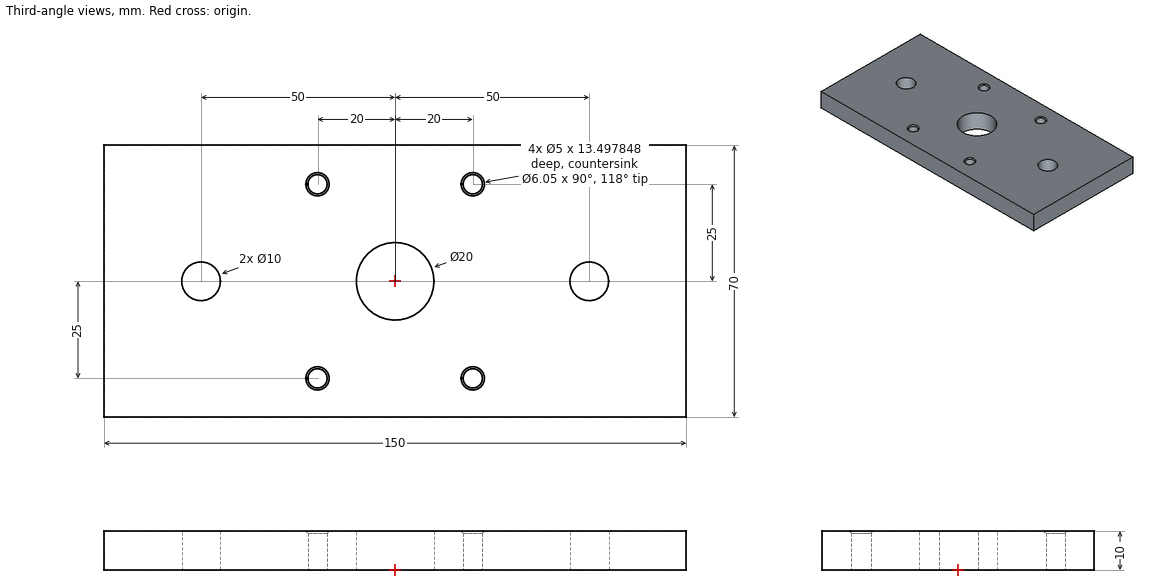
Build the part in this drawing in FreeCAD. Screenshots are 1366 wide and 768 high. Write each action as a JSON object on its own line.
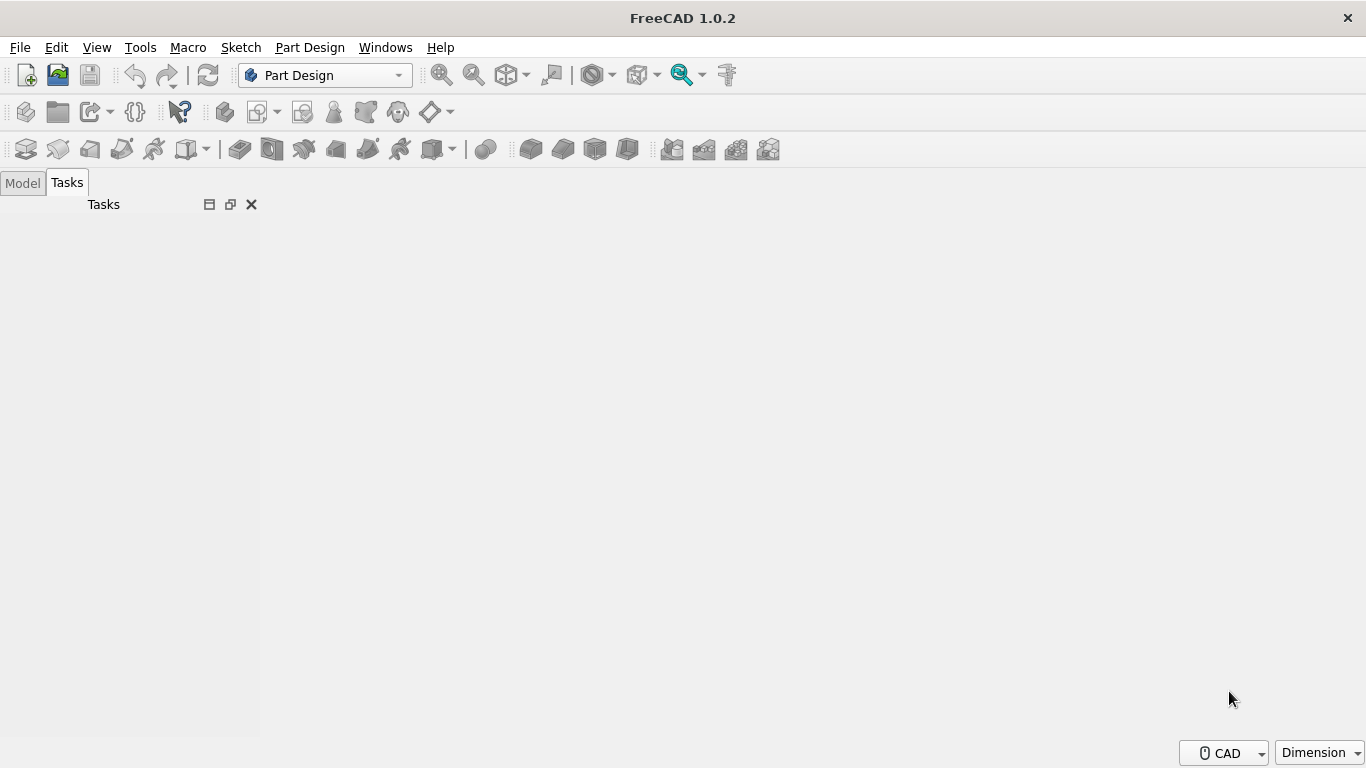
{"action": "left_click", "coordinate": [26, 76]}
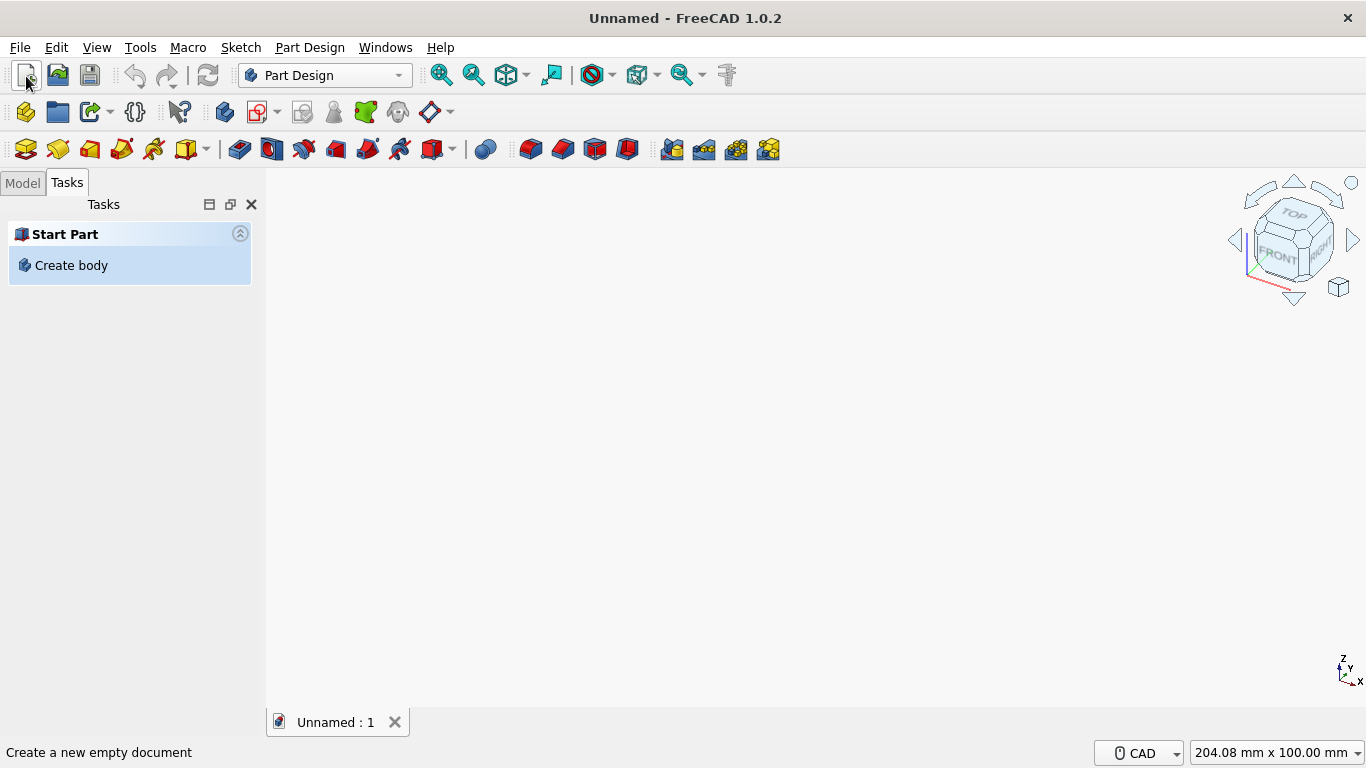
{"action": "left_click", "coordinate": [258, 112]}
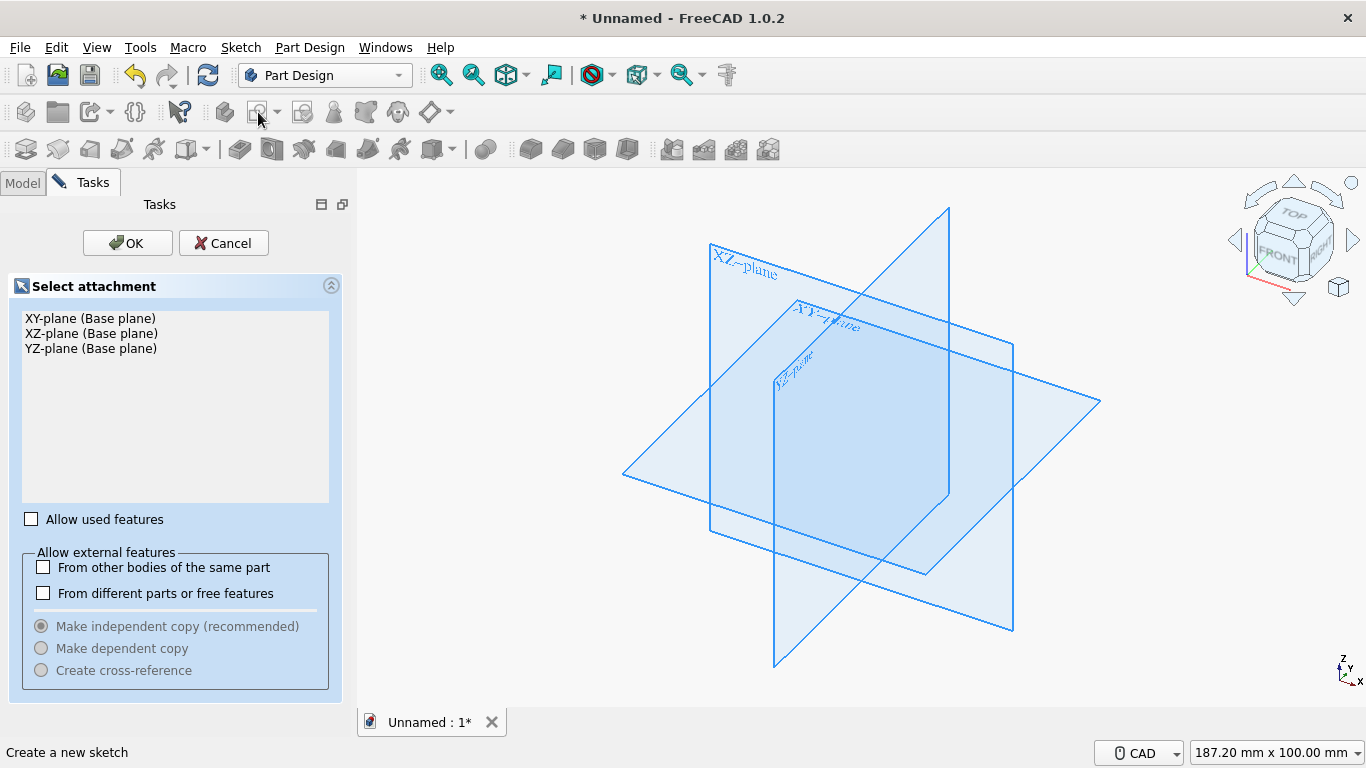
{"action": "left_click", "coordinate": [82, 318]}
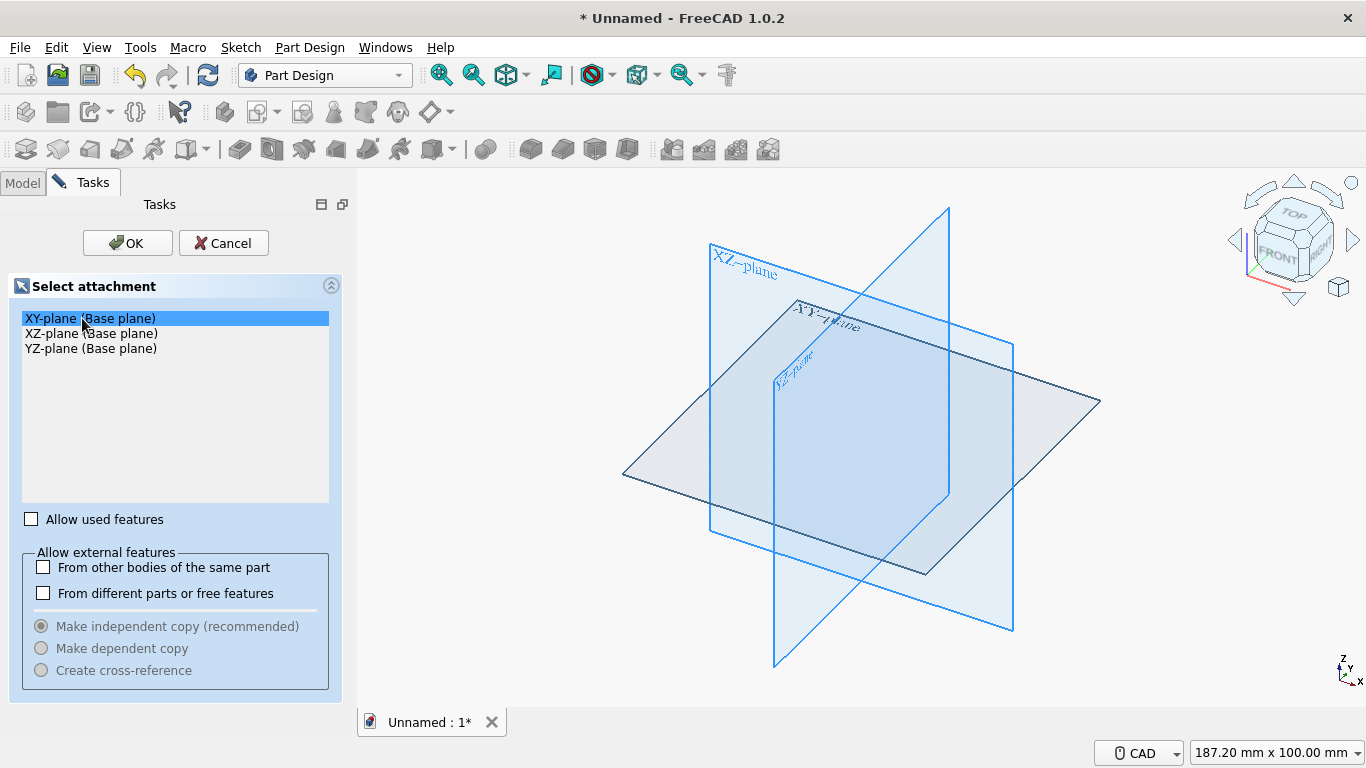
{"action": "left_click", "coordinate": [128, 243]}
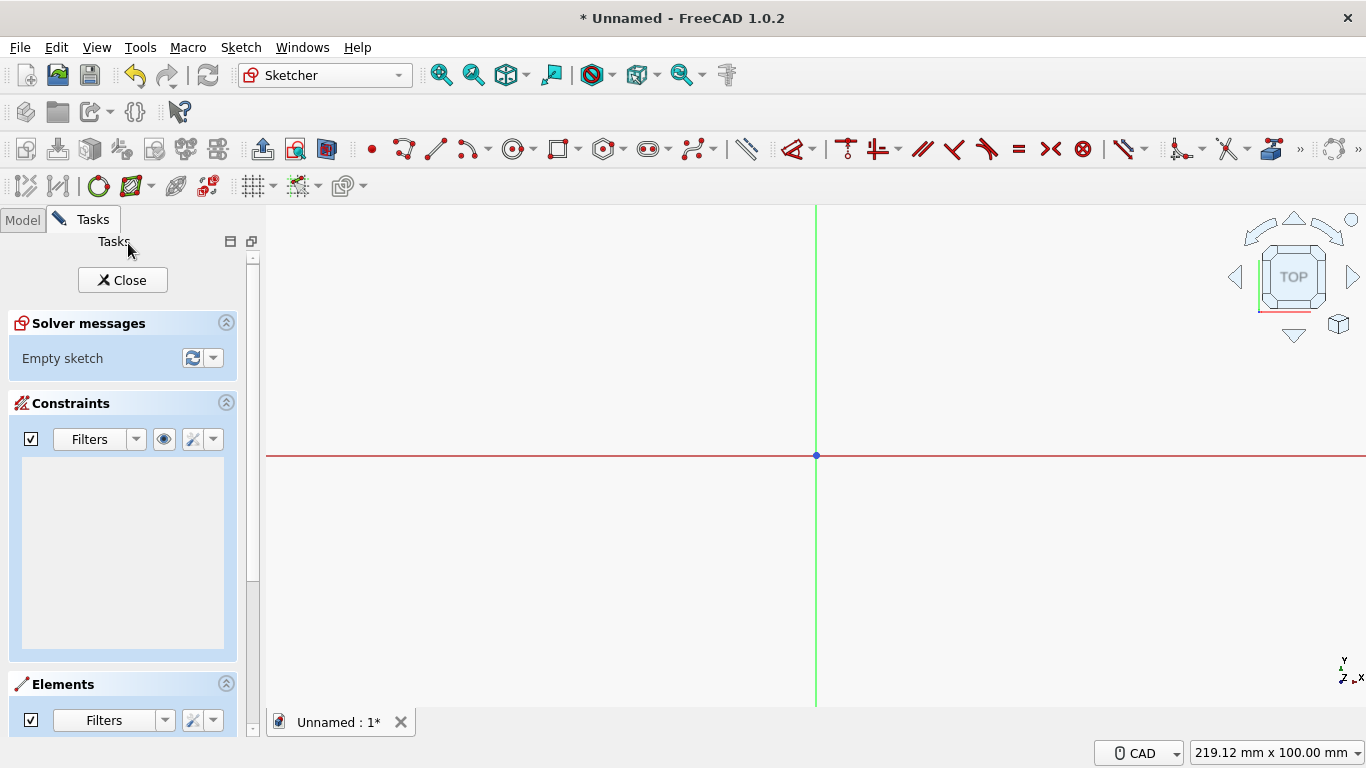
{"action": "scroll", "coordinate": [438, 456], "scroll_direction": "down", "scroll_amount": 1}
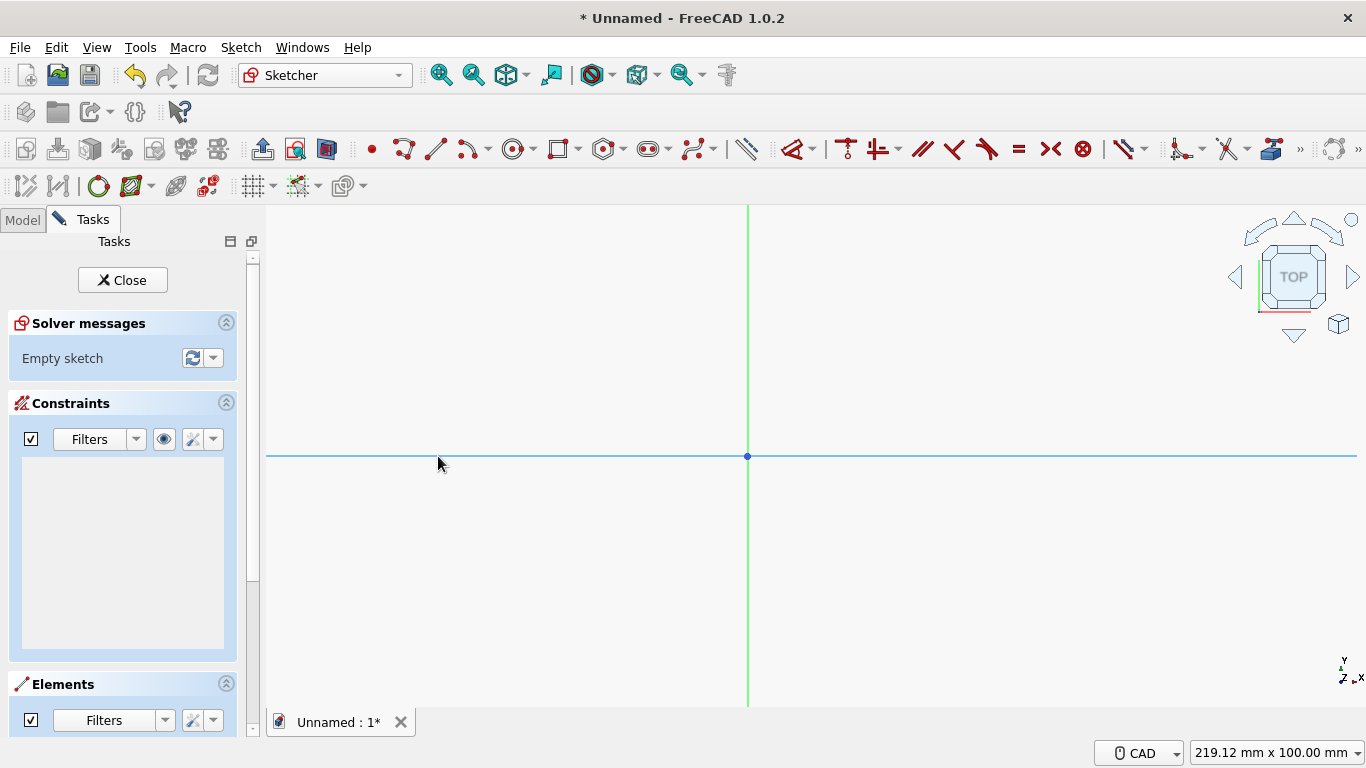
{"action": "left_click", "coordinate": [580, 150]}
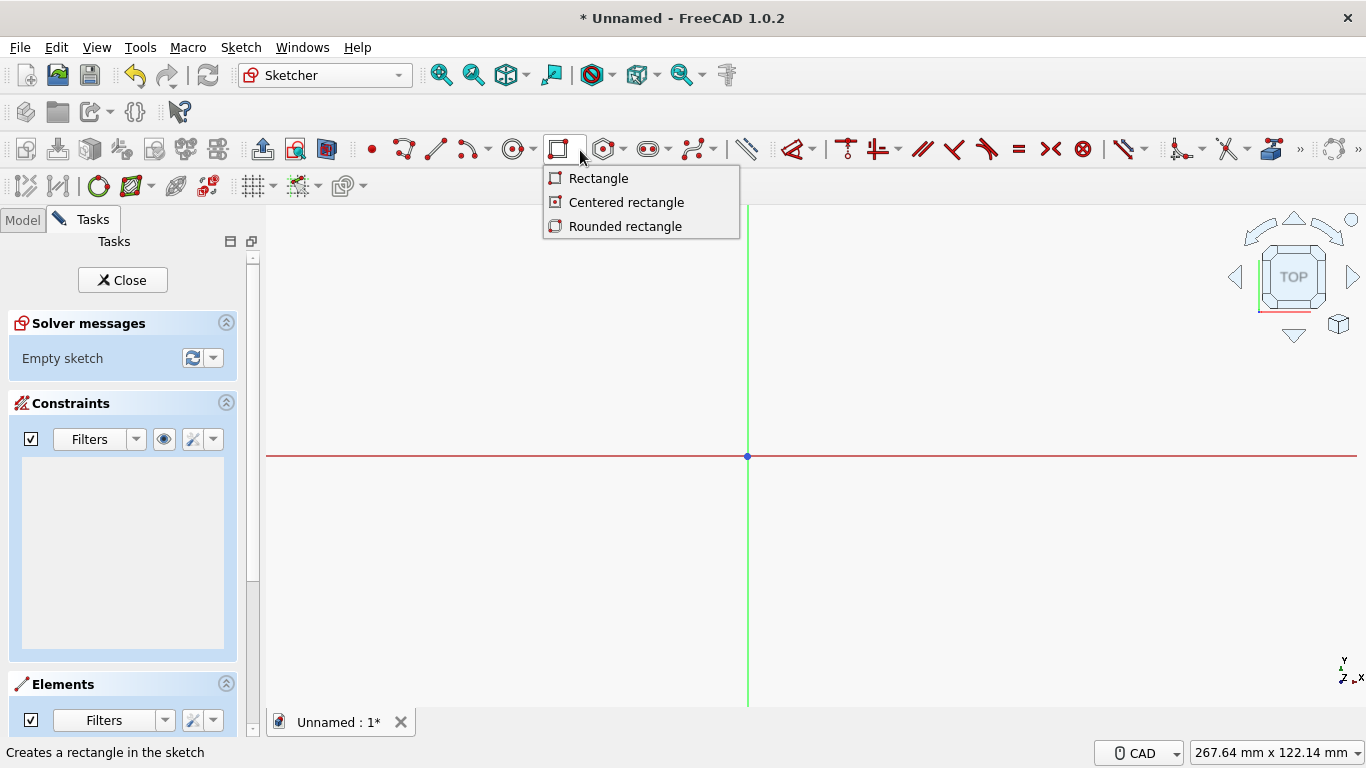
{"action": "left_click", "coordinate": [642, 202]}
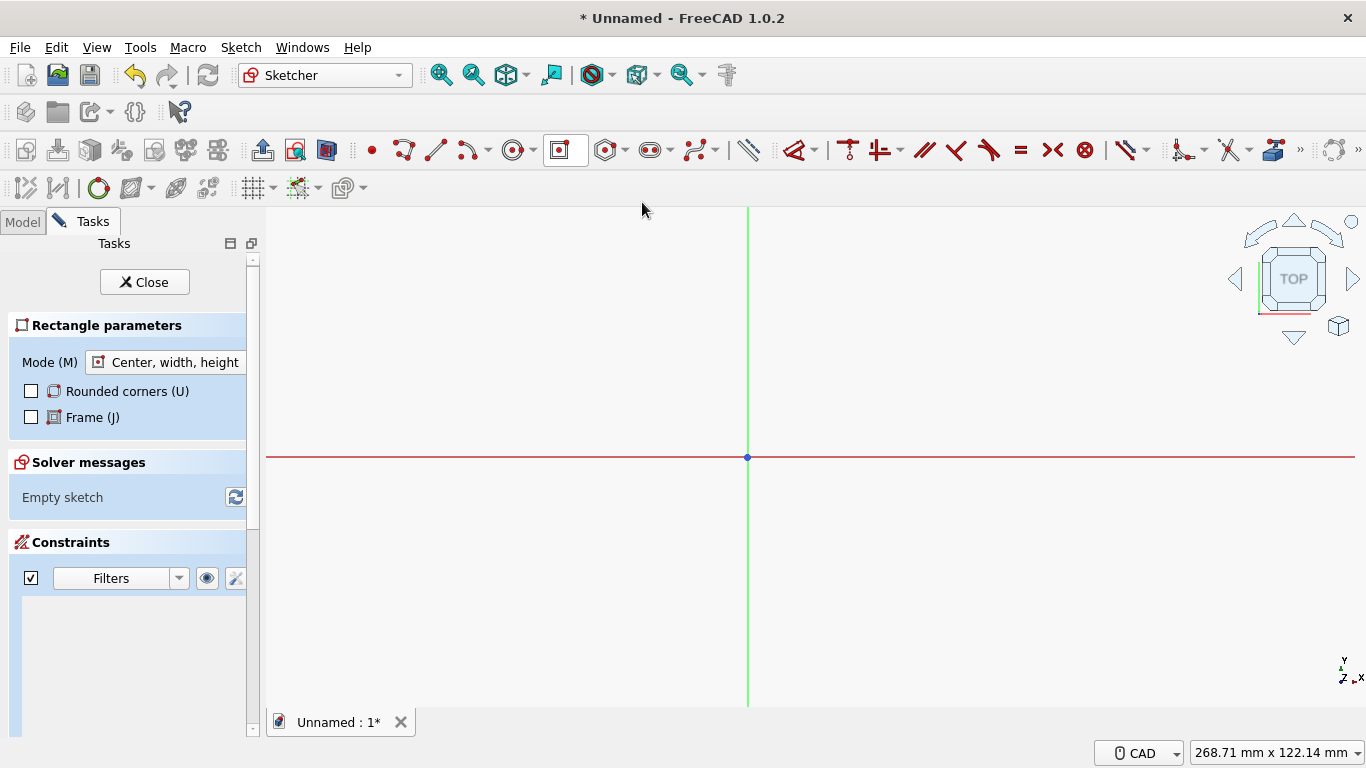
{"action": "left_click", "coordinate": [748, 457]}
{"action": "left_click", "coordinate": [1055, 314]}
{"action": "key", "text": "Escape"}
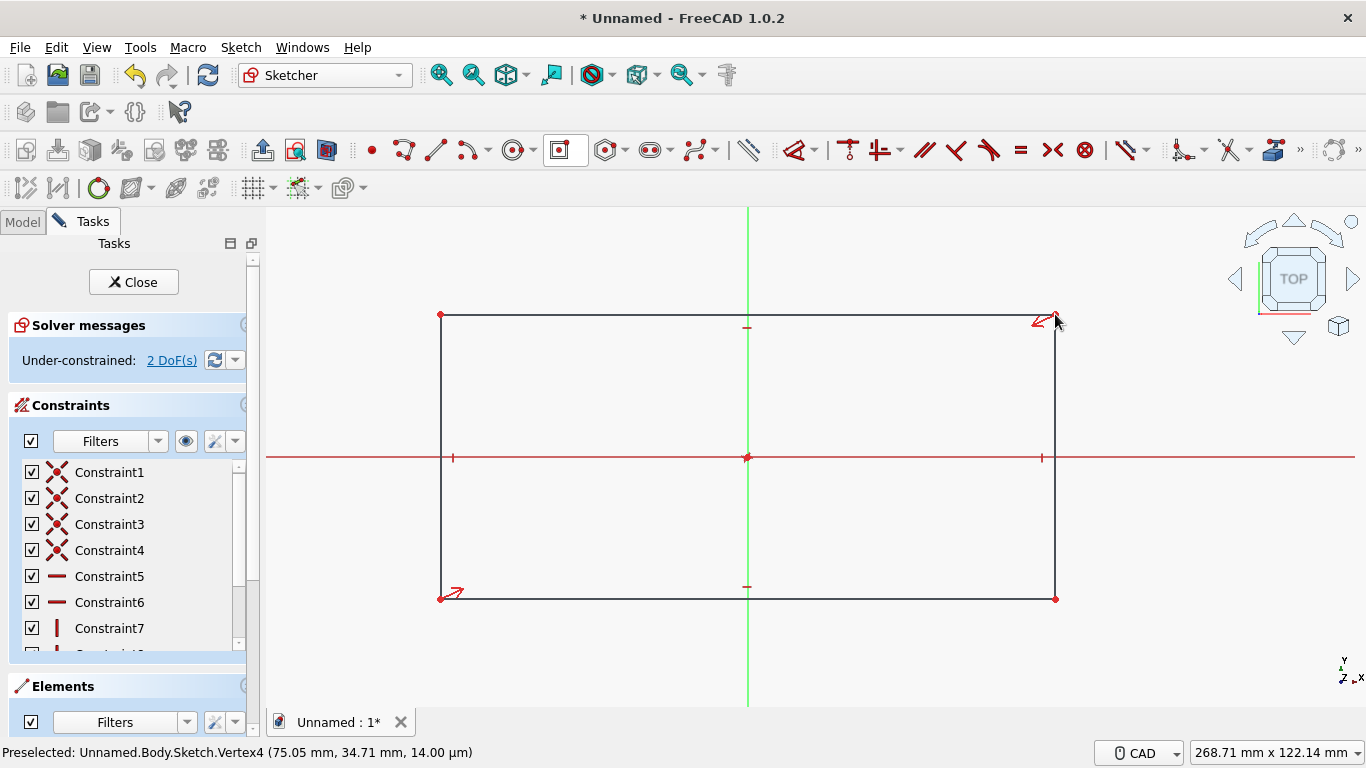
{"action": "left_click", "coordinate": [1055, 514]}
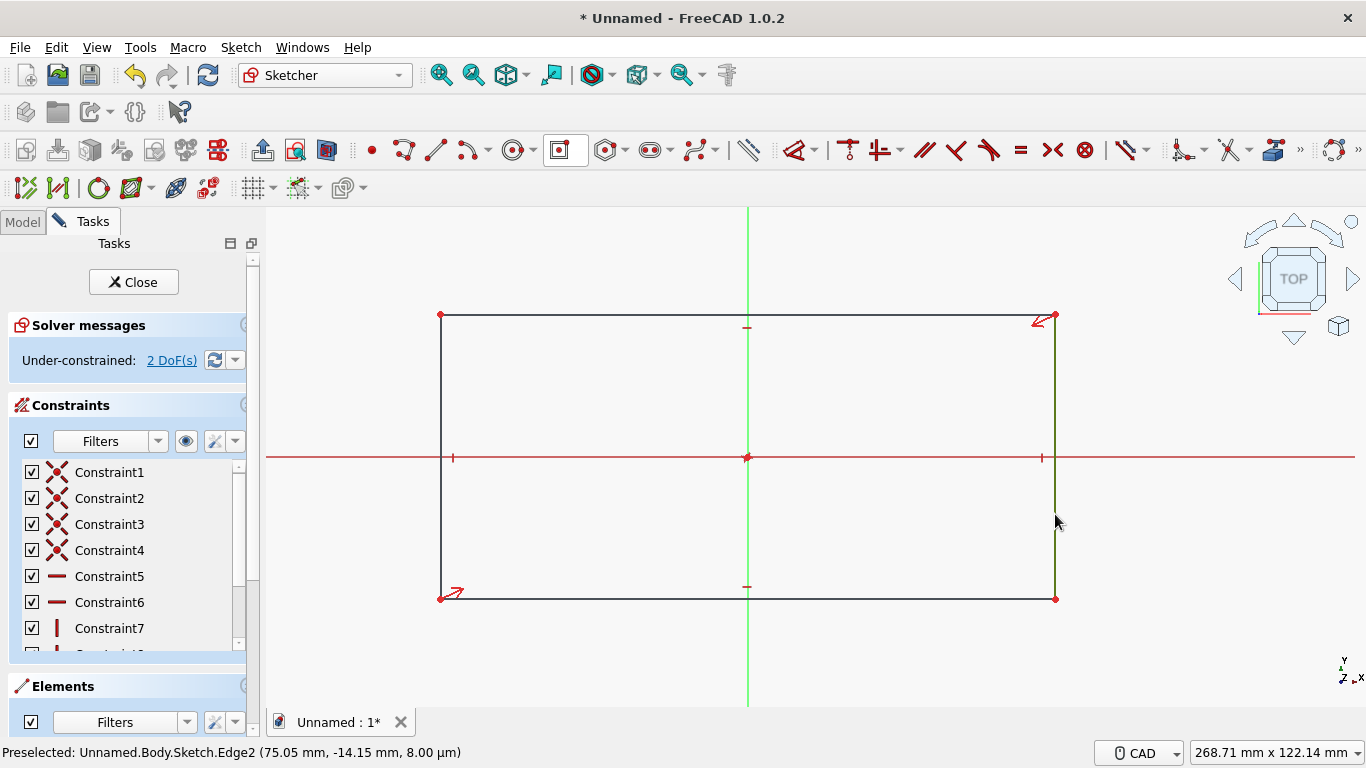
{"action": "left_click", "coordinate": [816, 150]}